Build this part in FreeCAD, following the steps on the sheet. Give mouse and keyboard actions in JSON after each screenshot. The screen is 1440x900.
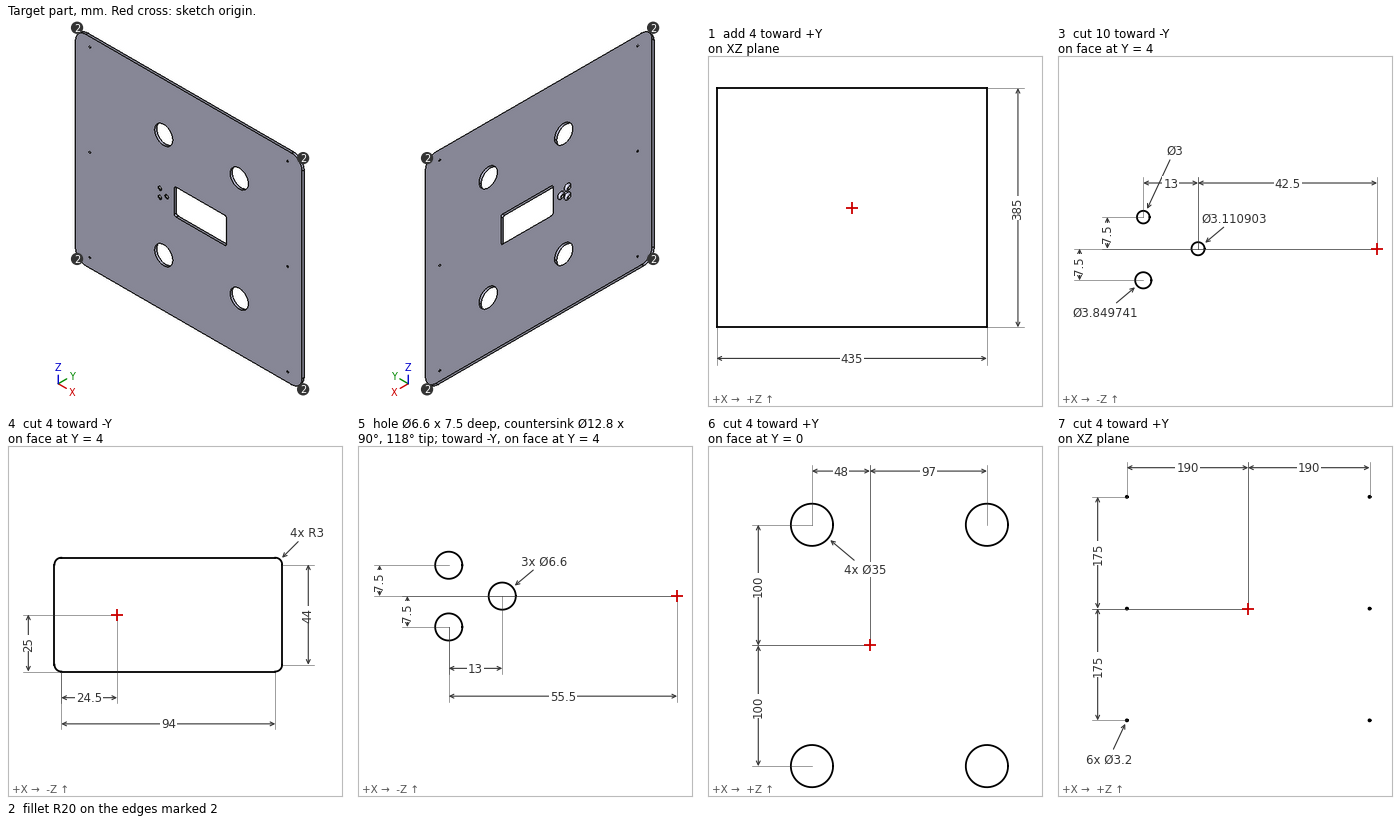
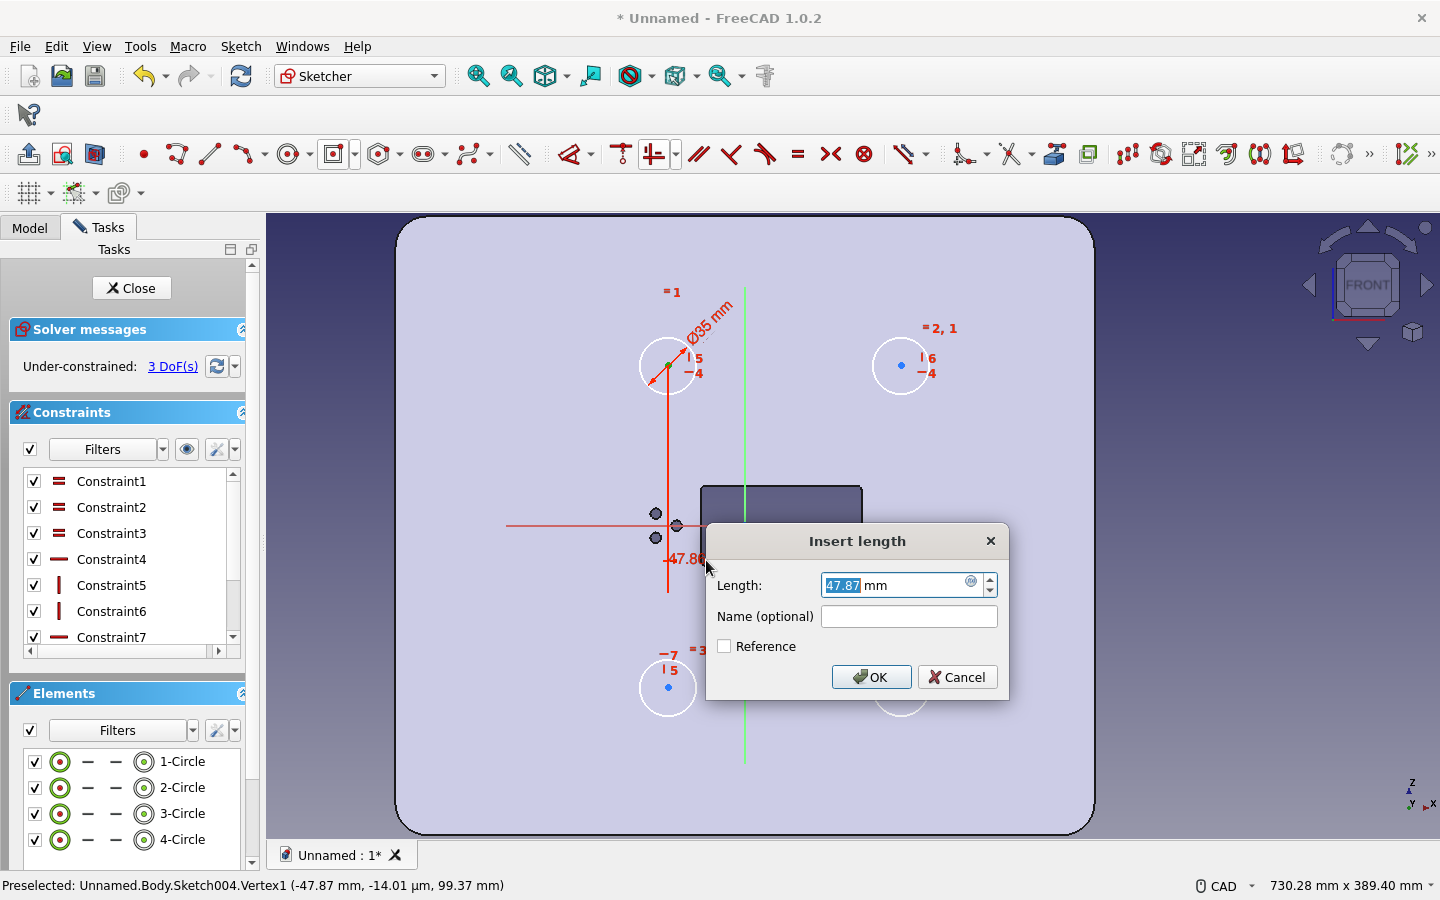
{"action": "type", "text": "48"}
{"action": "key", "text": "Return"}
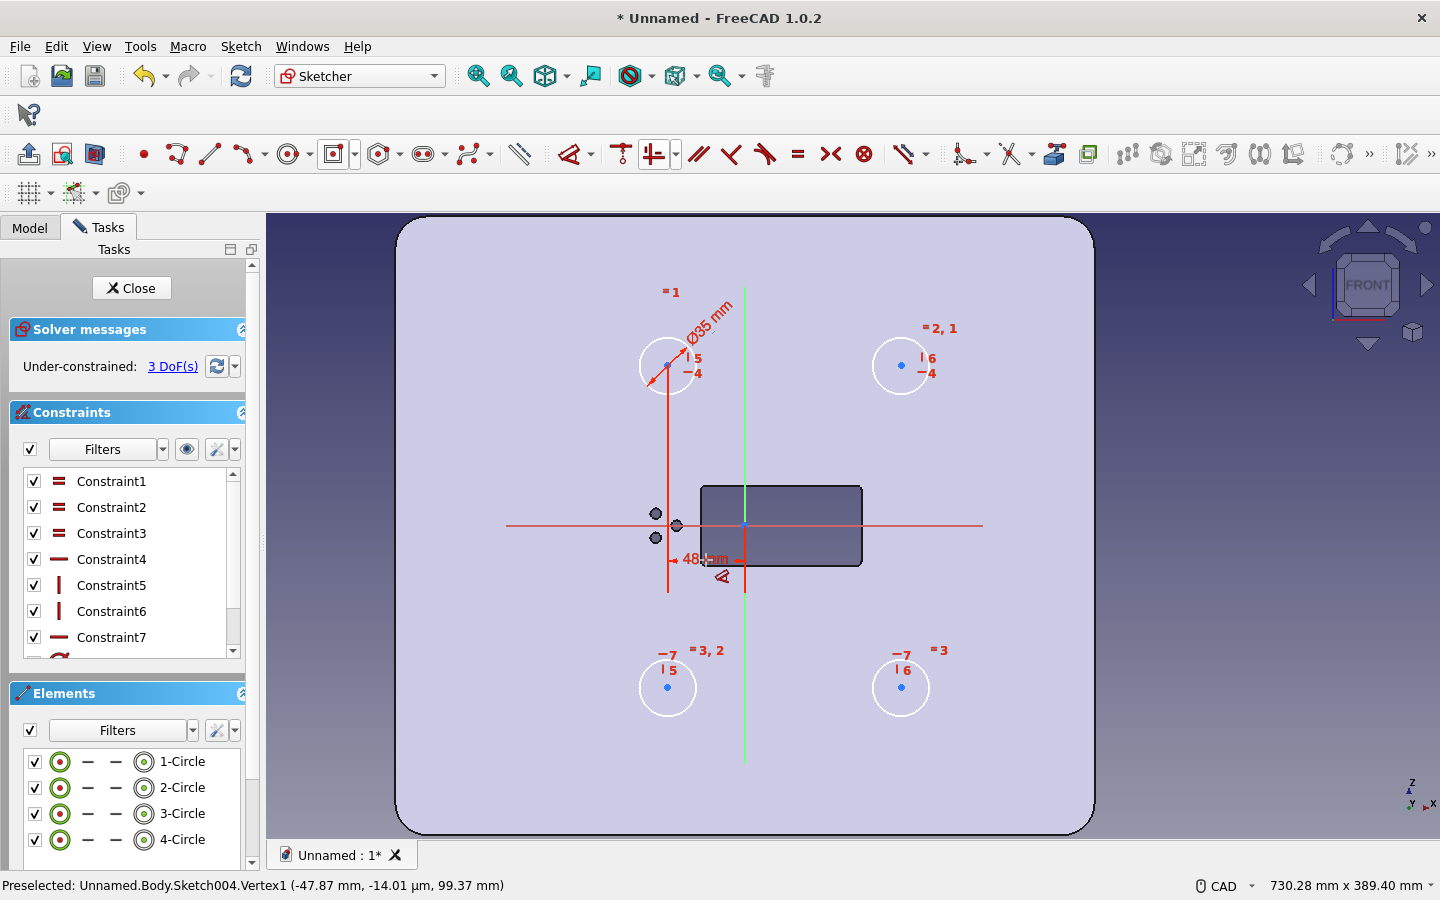
{"action": "left_click", "coordinate": [901, 366]}
{"action": "left_click", "coordinate": [823, 332]}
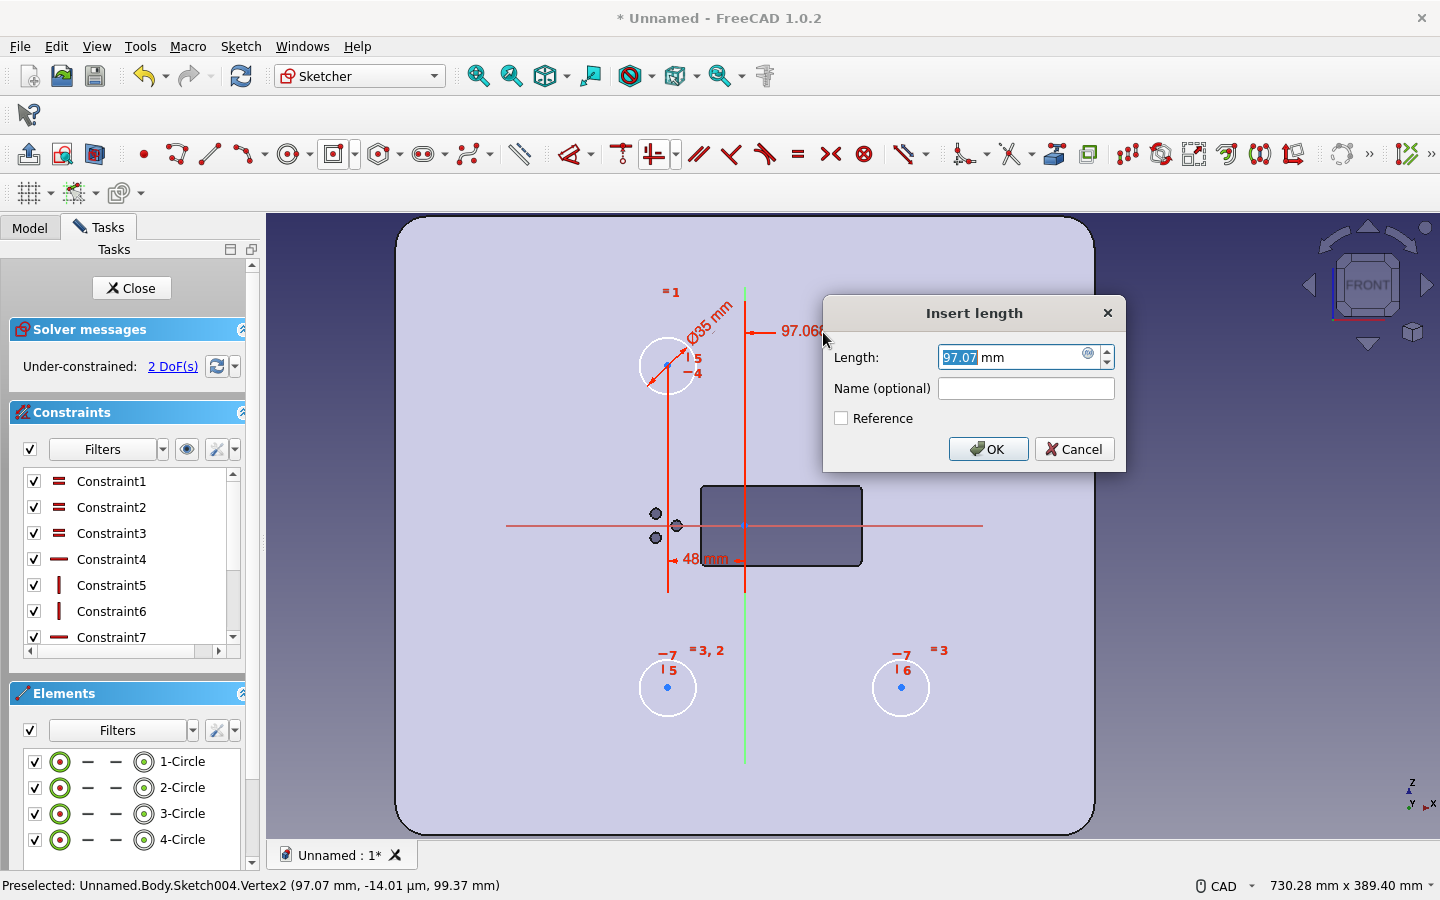
{"action": "type", "text": "97"}
{"action": "key", "text": "Return"}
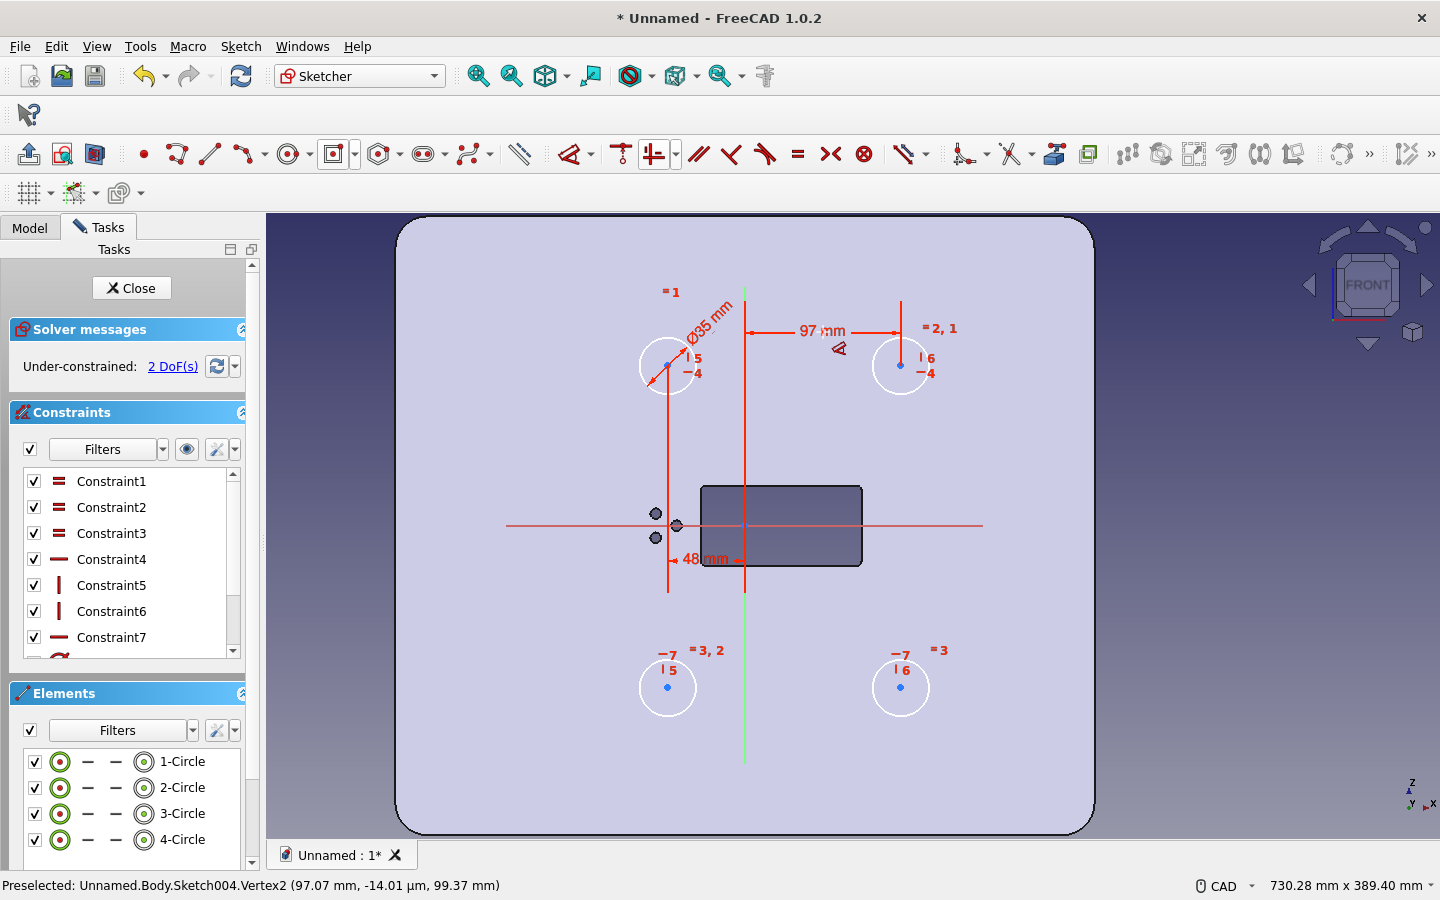
{"action": "left_click", "coordinate": [668, 366]}
{"action": "left_click", "coordinate": [634, 446]}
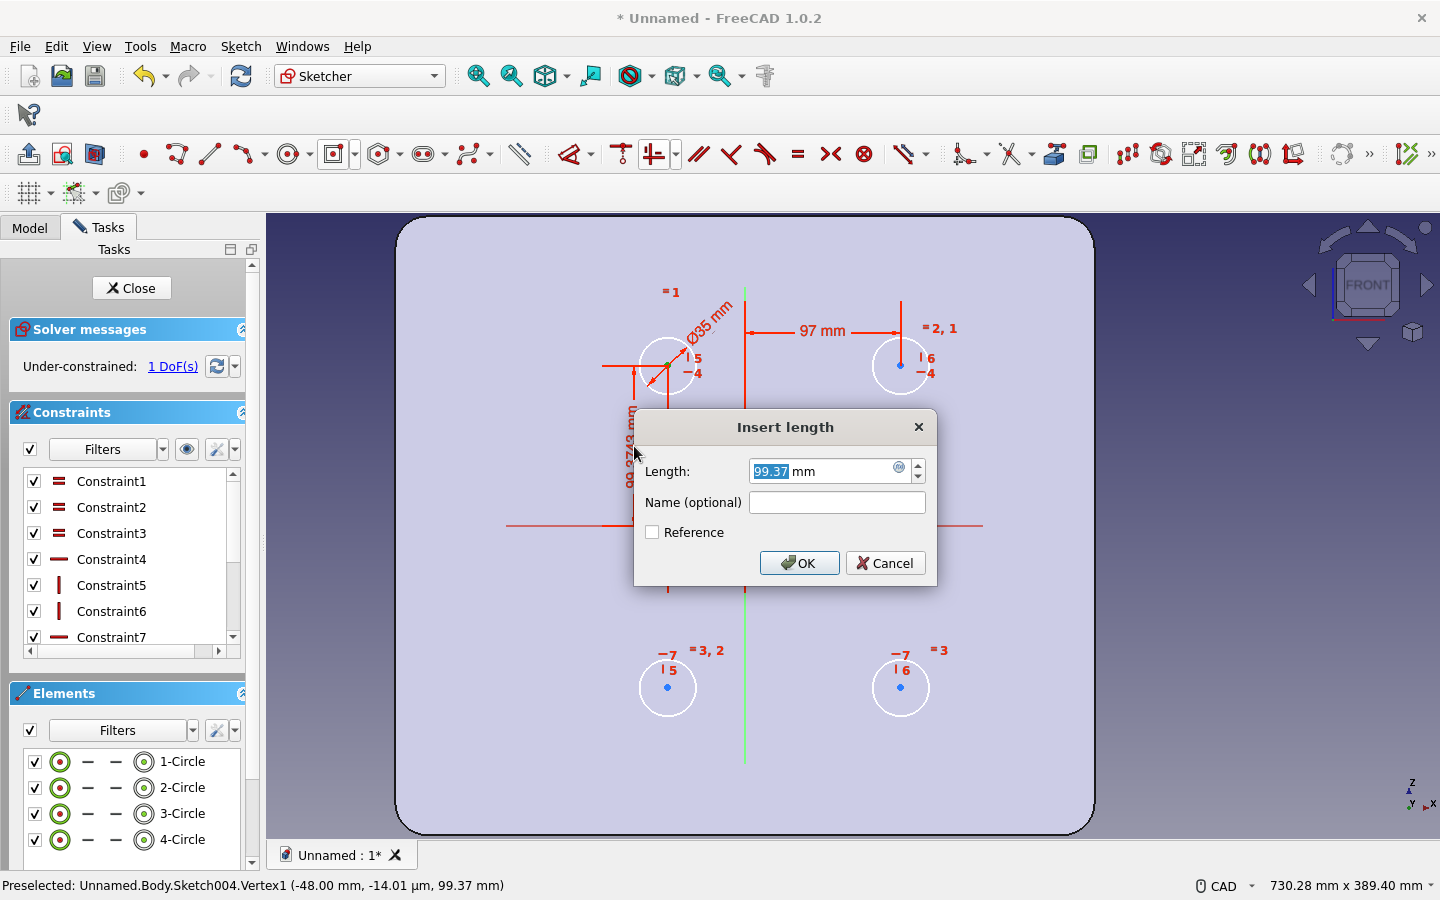
{"action": "type", "text": "100"}
{"action": "key", "text": "Return"}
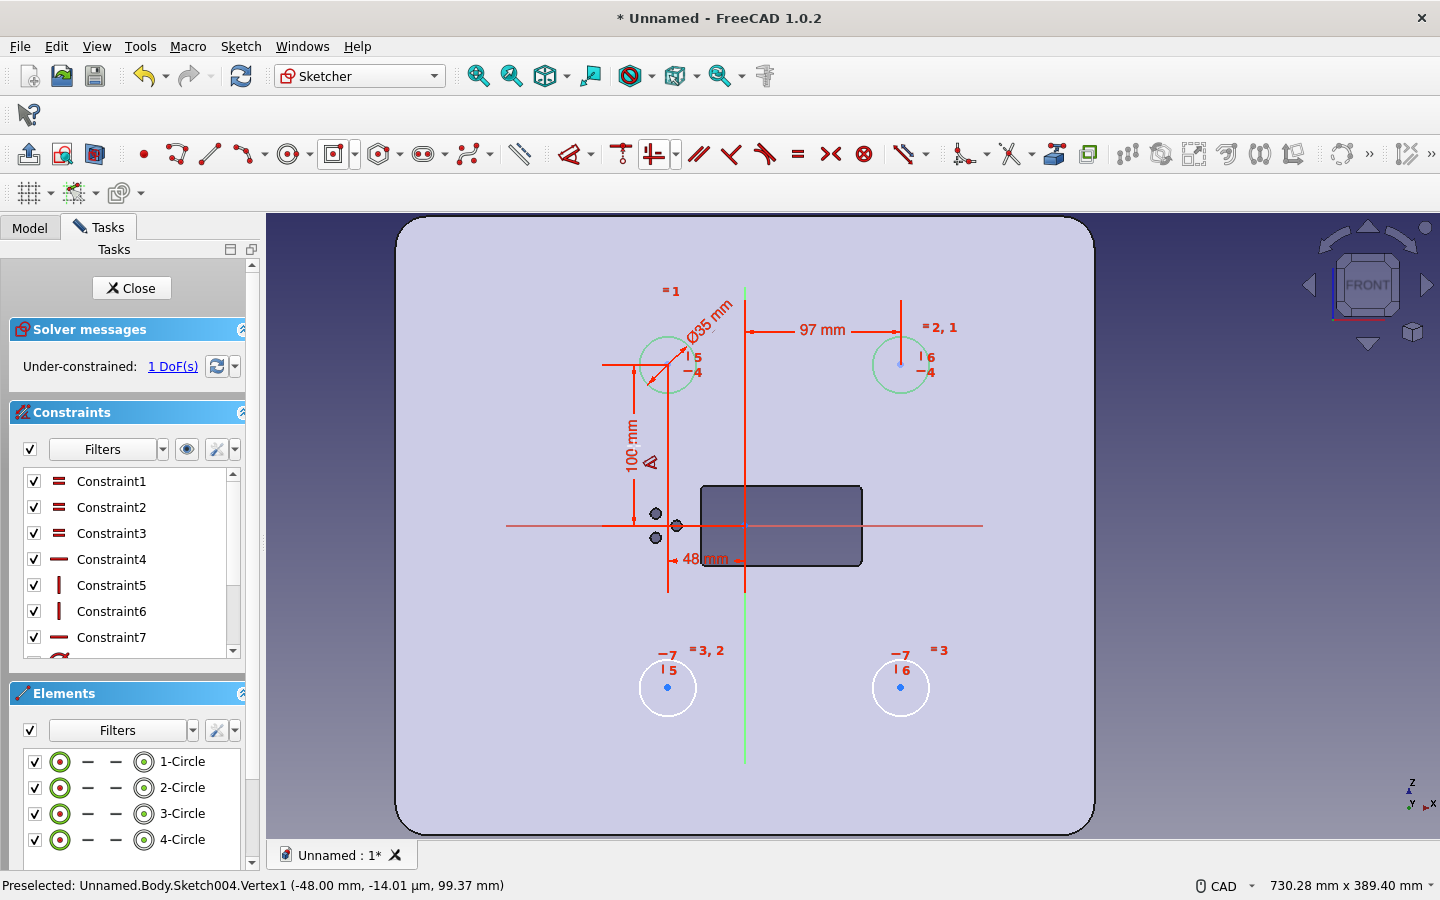
{"action": "left_click", "coordinate": [668, 688]}
{"action": "left_click", "coordinate": [634, 607]}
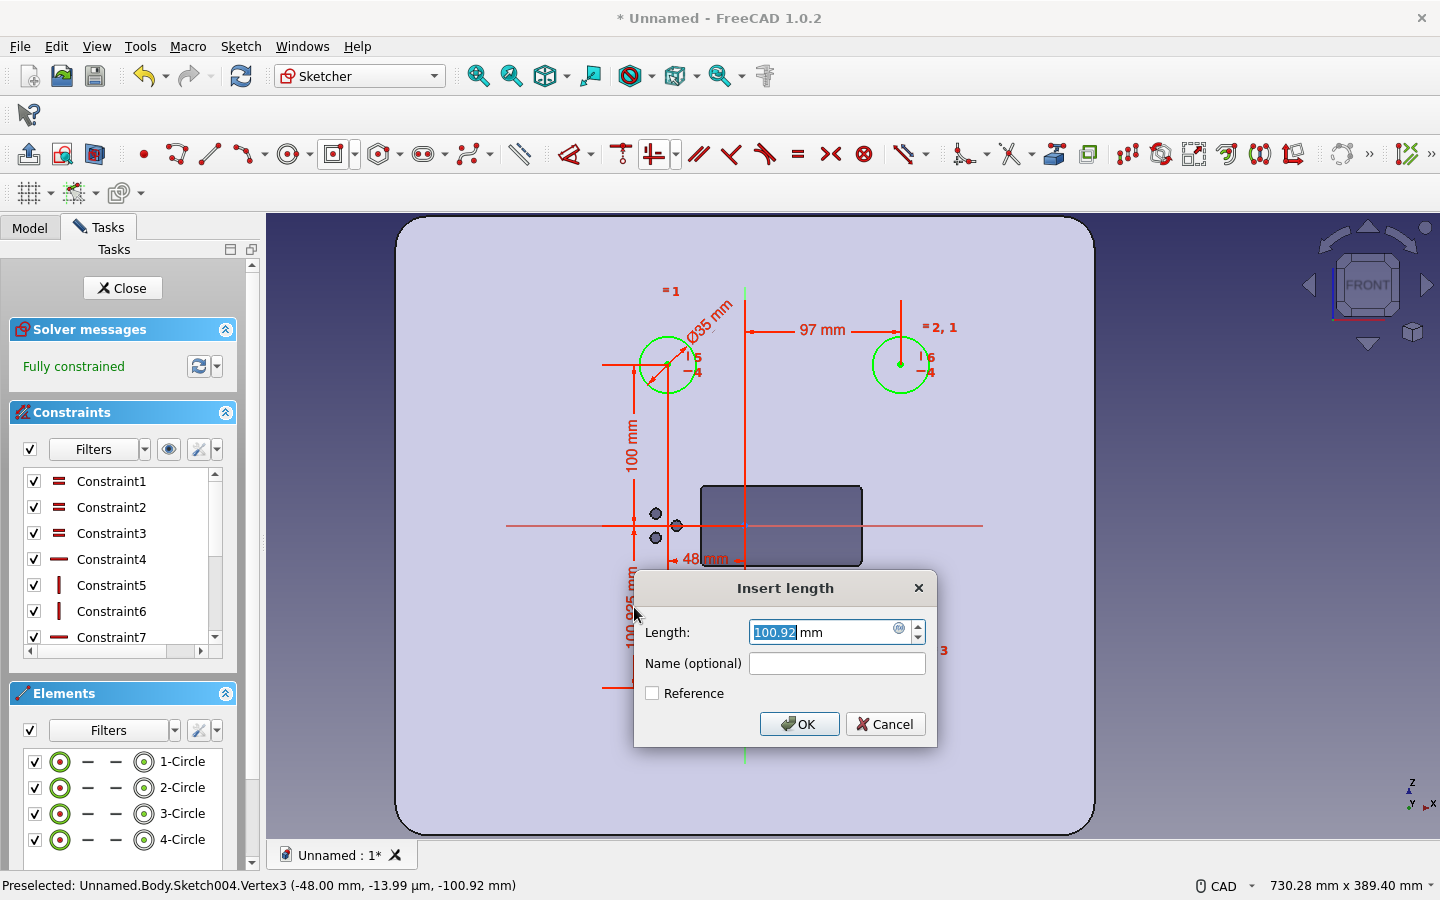
{"action": "type", "text": "100"}
{"action": "key", "text": "Return"}
{"action": "key", "text": "Escape"}